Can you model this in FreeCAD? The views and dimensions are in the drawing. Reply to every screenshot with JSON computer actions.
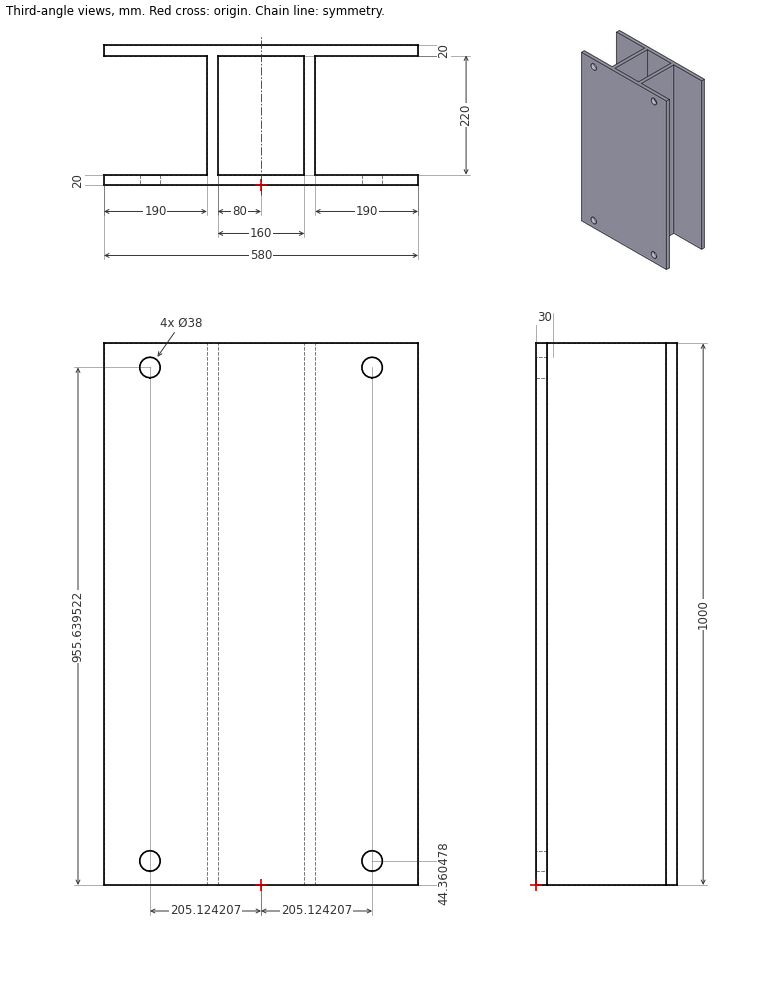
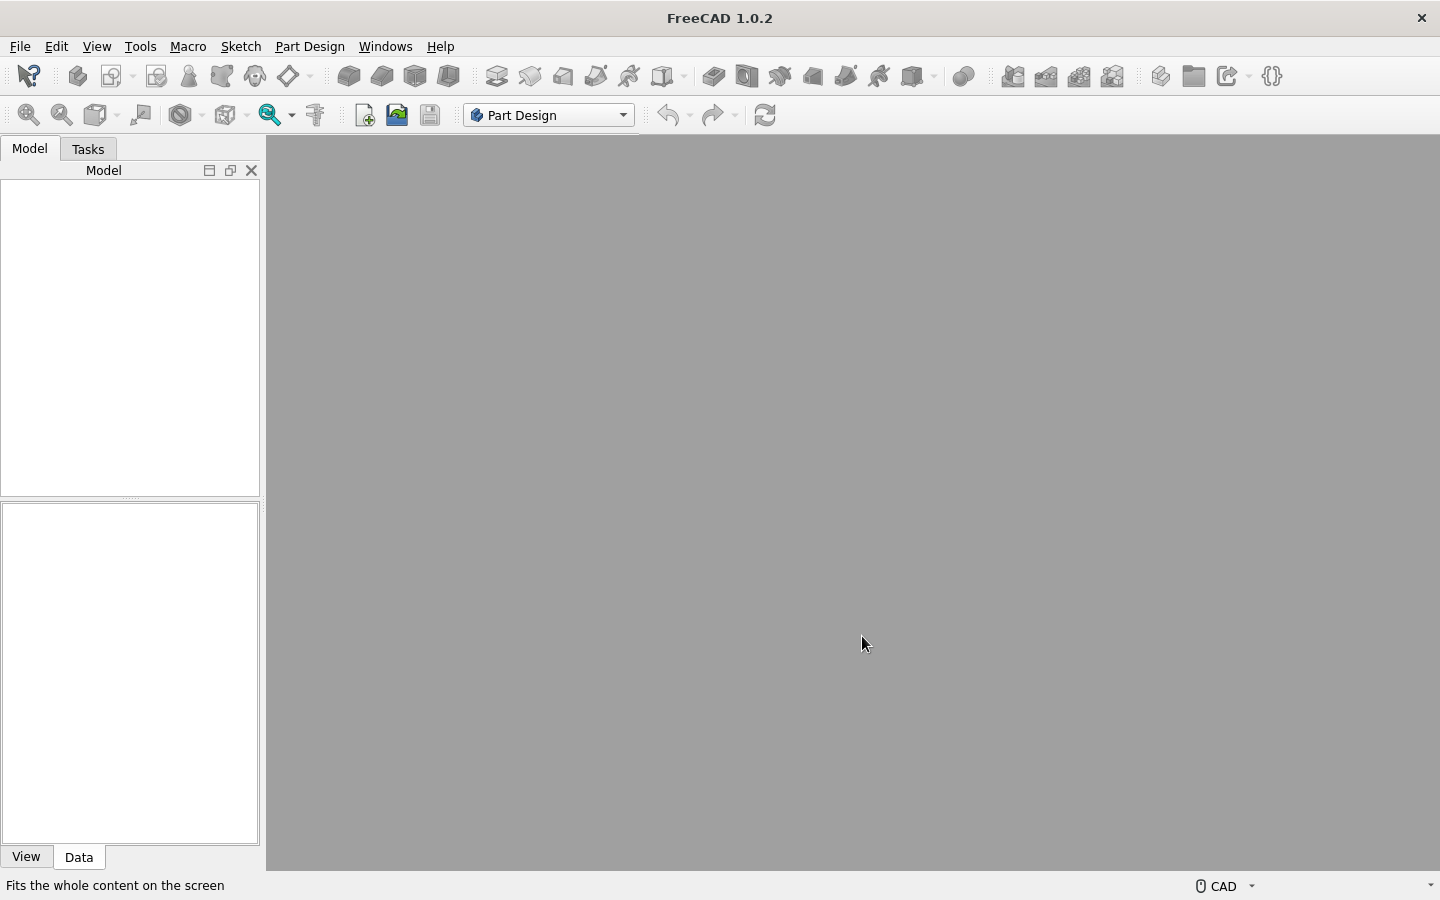
{"action": "key", "text": "ctrl+n"}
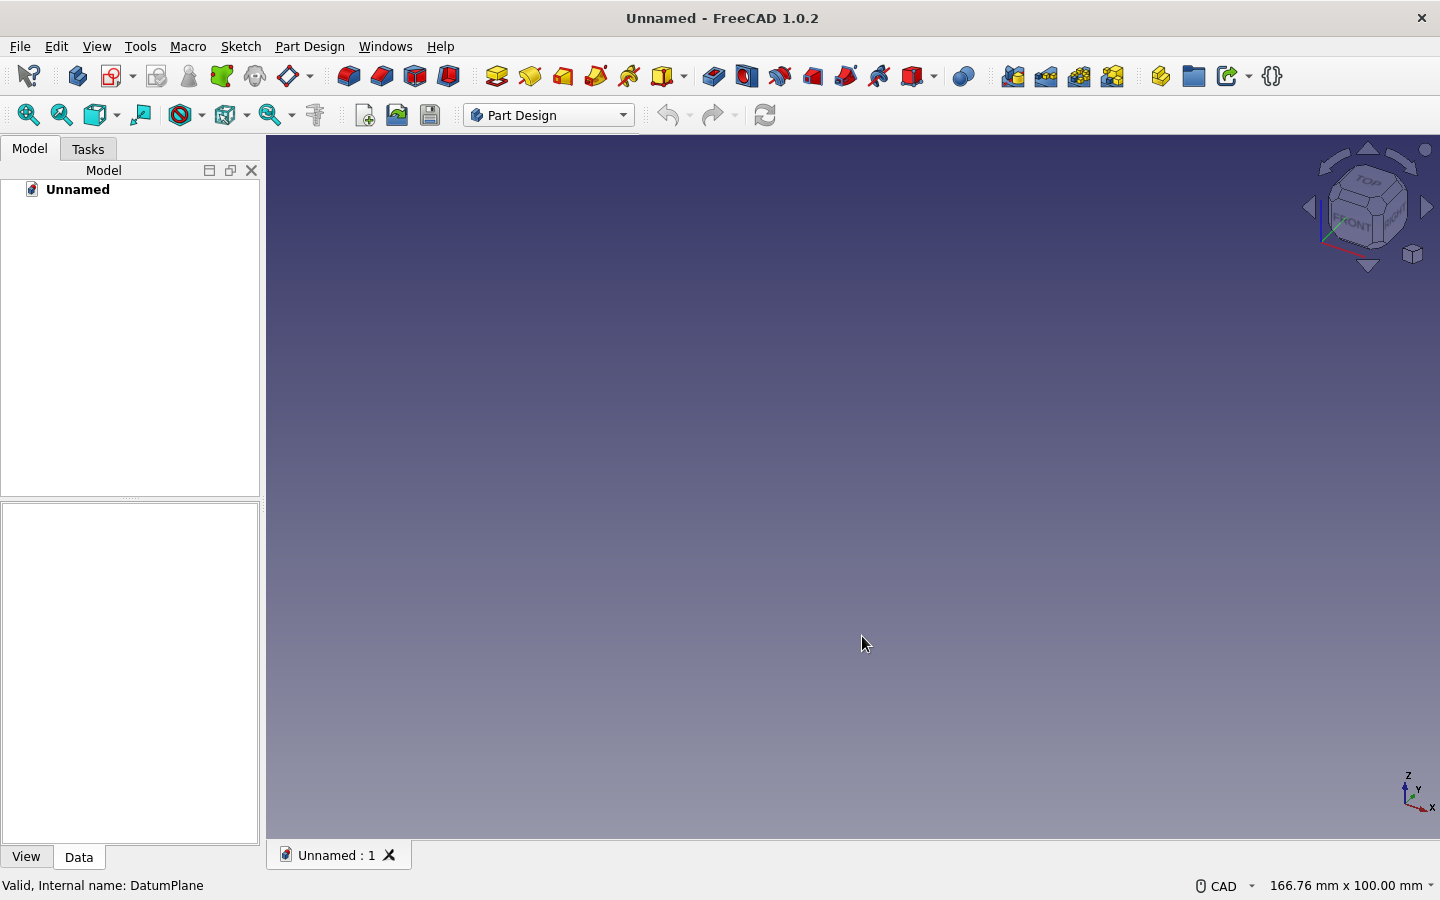
{"action": "left_click", "coordinate": [110, 76]}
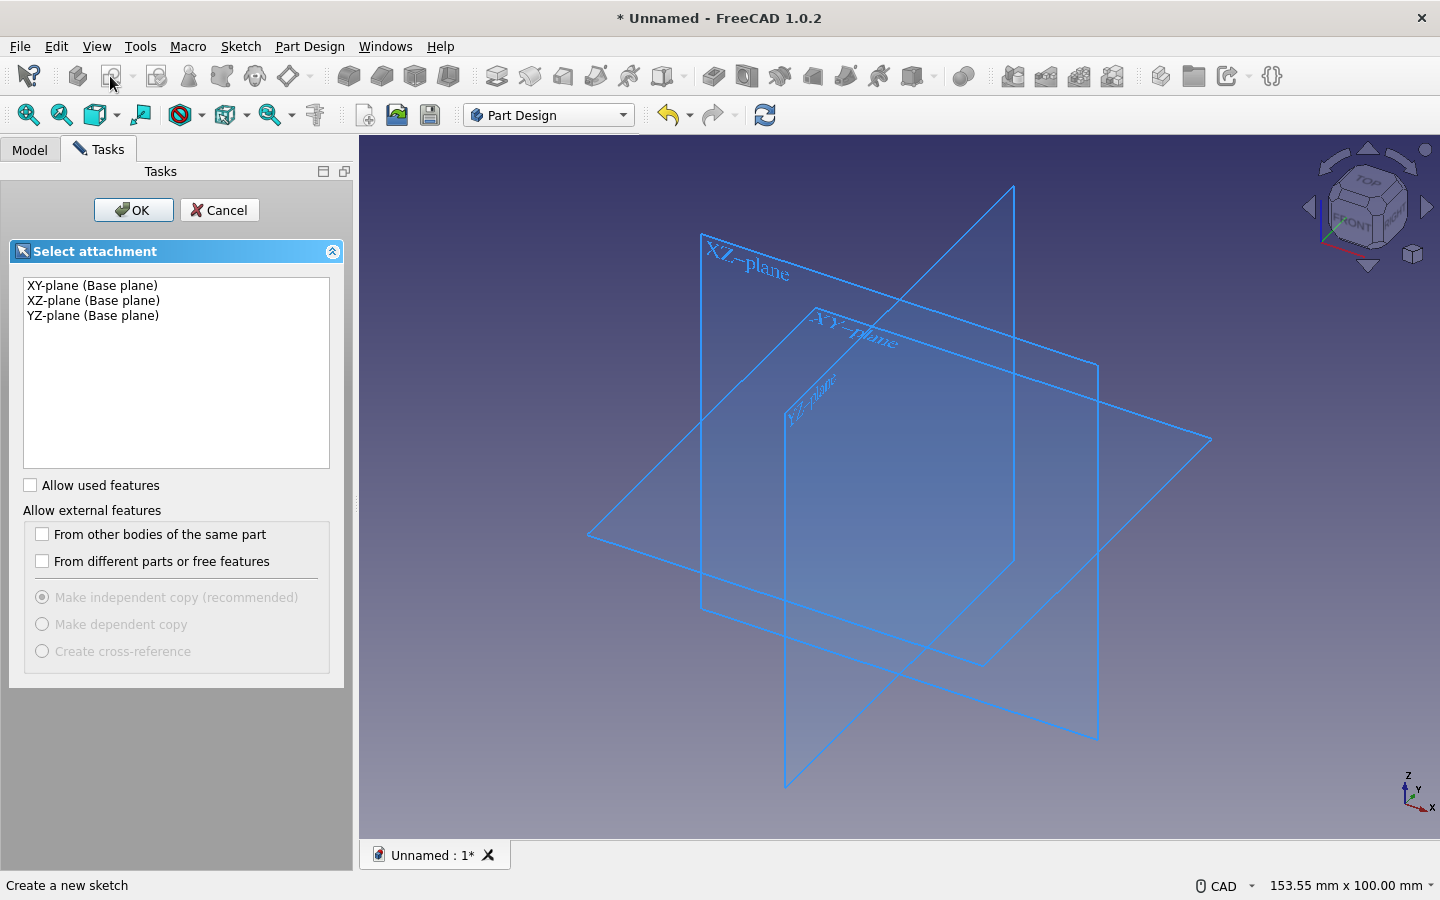
{"action": "left_click", "coordinate": [84, 286]}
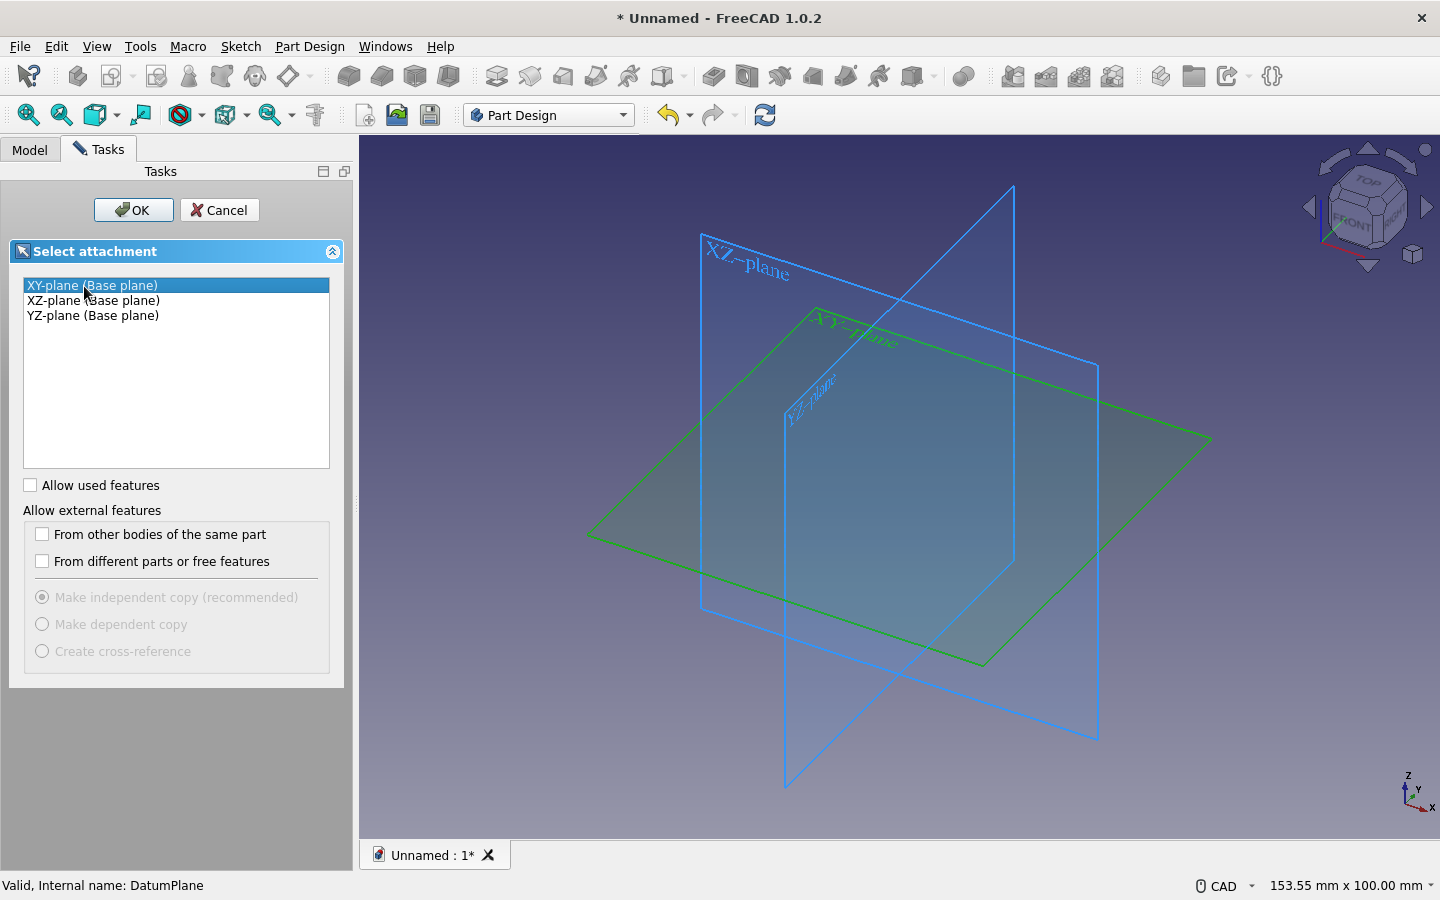
{"action": "left_click", "coordinate": [134, 210]}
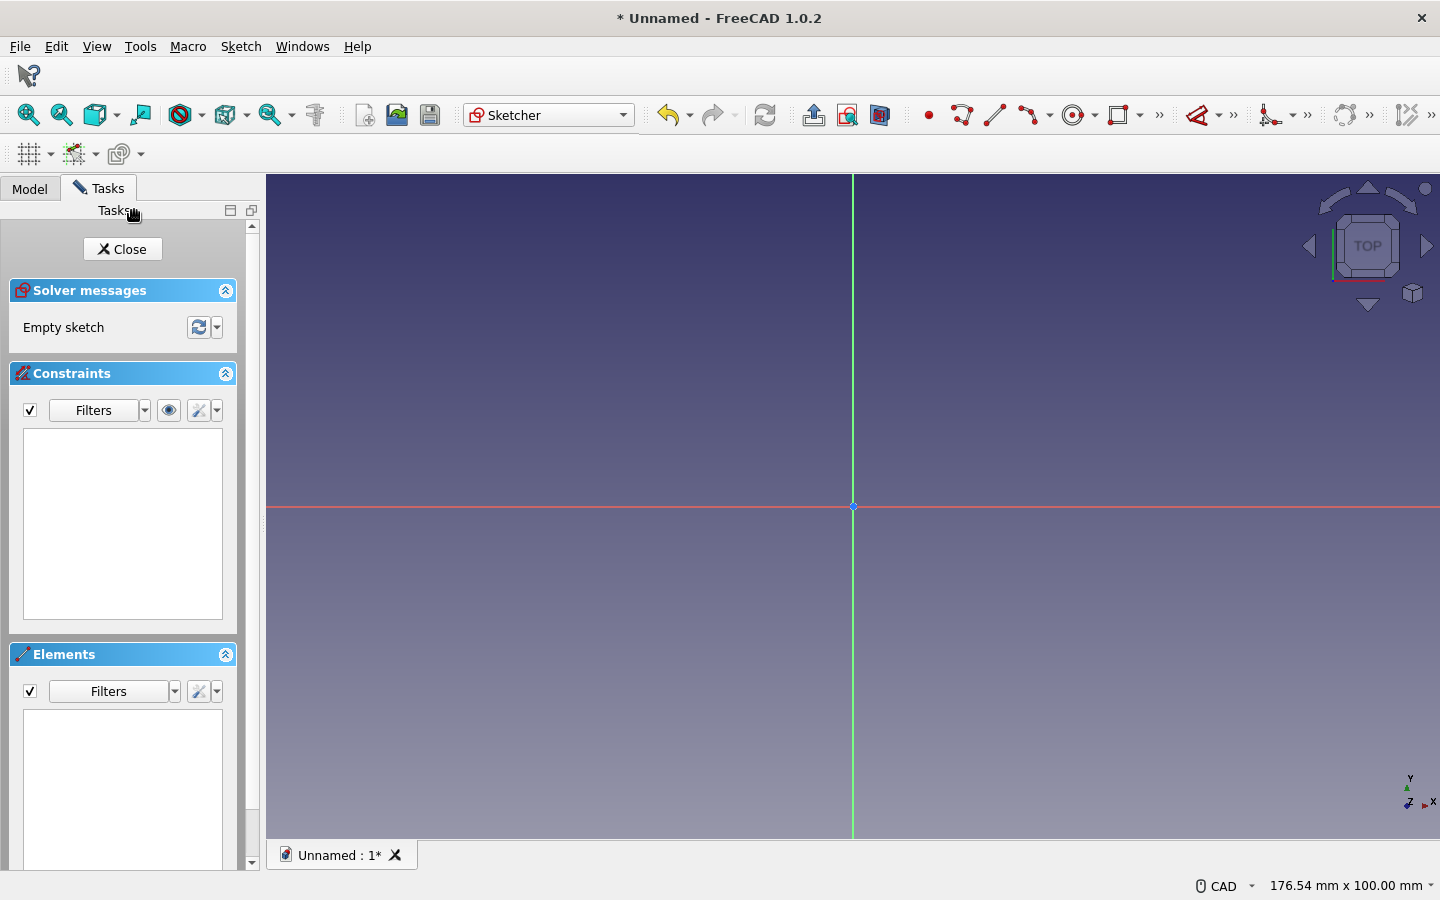
{"action": "scroll", "coordinate": [771, 678], "scroll_direction": "down", "scroll_amount": 9}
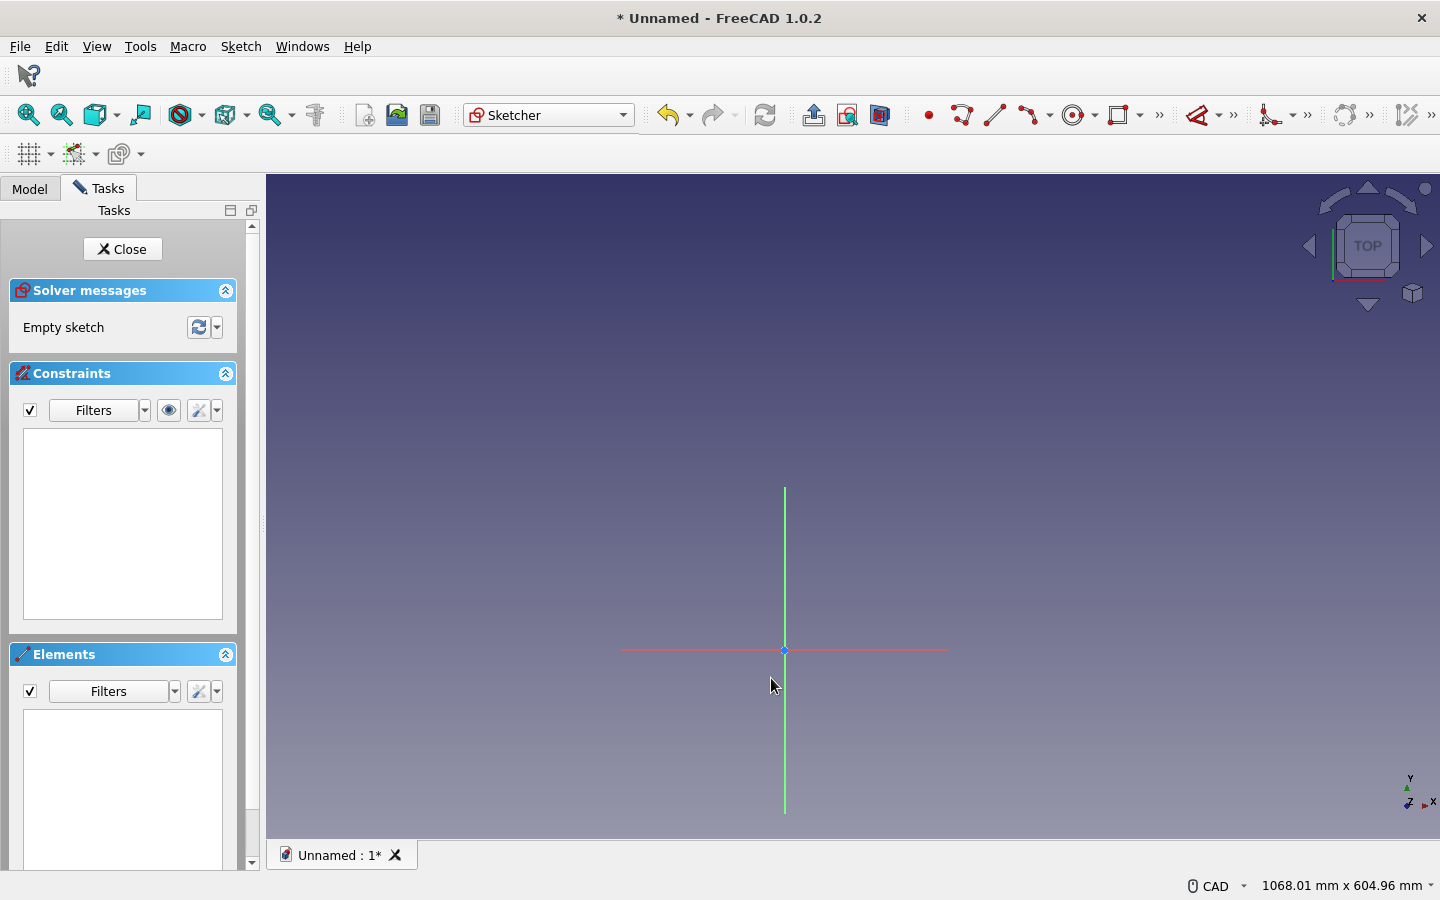
{"action": "left_click", "coordinate": [962, 116]}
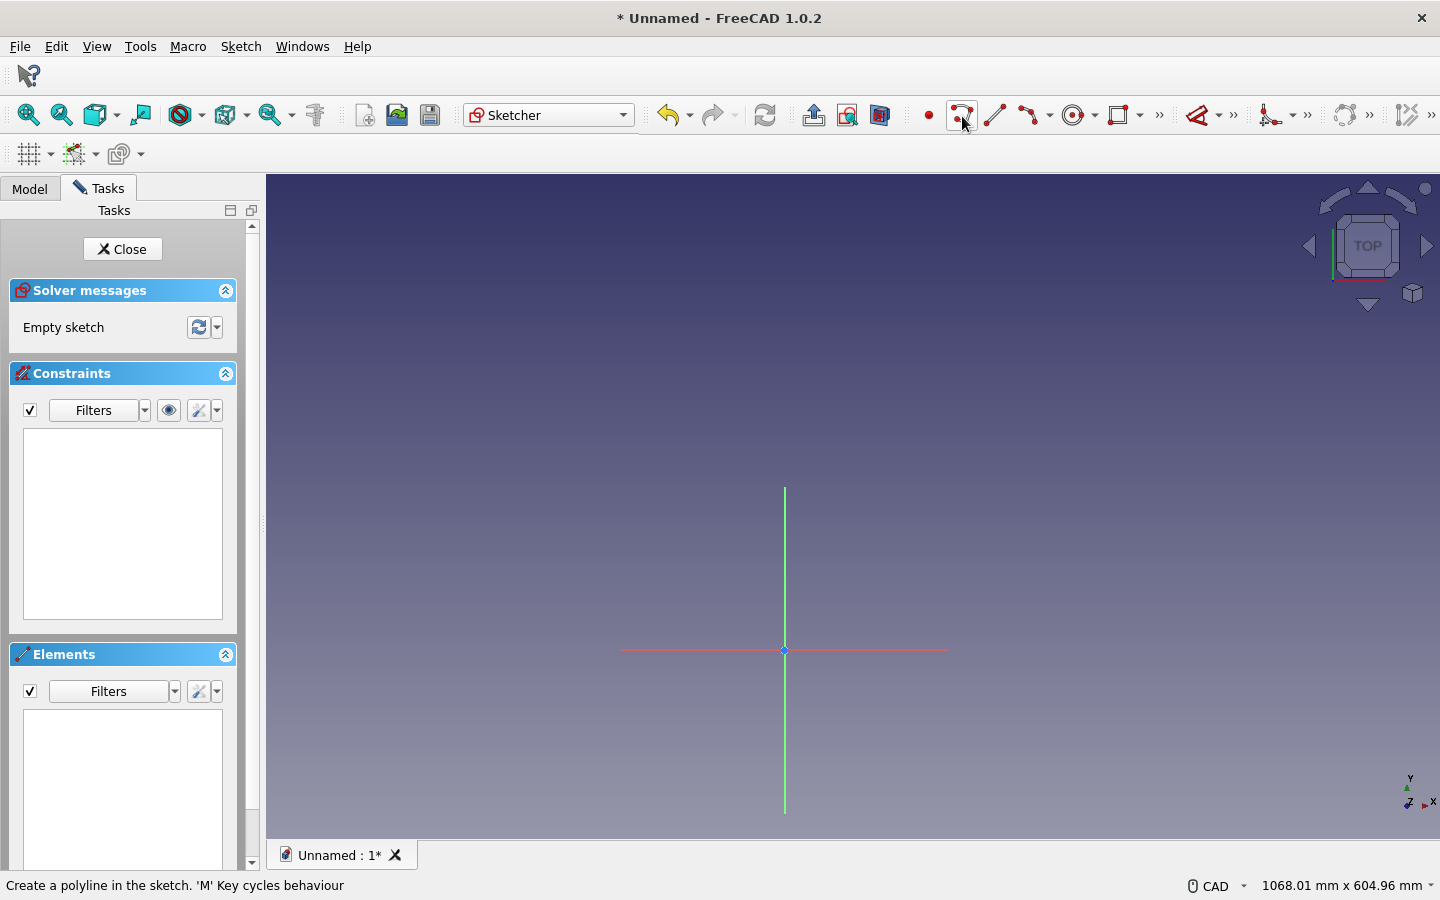
{"action": "left_click", "coordinate": [675, 628]}
{"action": "left_click", "coordinate": [466, 628]}
{"action": "left_click", "coordinate": [466, 650]}
{"action": "left_click", "coordinate": [1104, 641]}
{"action": "left_click", "coordinate": [1104, 628]}
{"action": "left_click", "coordinate": [895, 628]}
{"action": "left_click", "coordinate": [895, 386]}
{"action": "left_click", "coordinate": [1104, 386]}
{"action": "left_click", "coordinate": [1104, 364]}
{"action": "left_click", "coordinate": [466, 364]}
{"action": "left_click", "coordinate": [466, 386]}
{"action": "left_click", "coordinate": [675, 386]}
{"action": "left_click", "coordinate": [675, 629]}